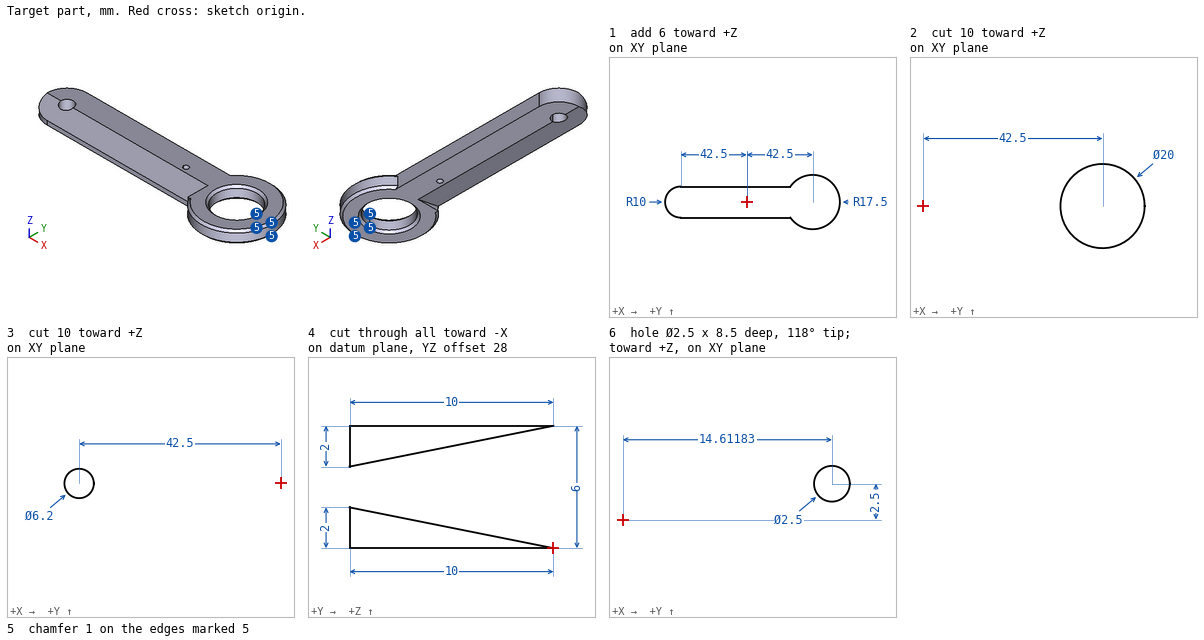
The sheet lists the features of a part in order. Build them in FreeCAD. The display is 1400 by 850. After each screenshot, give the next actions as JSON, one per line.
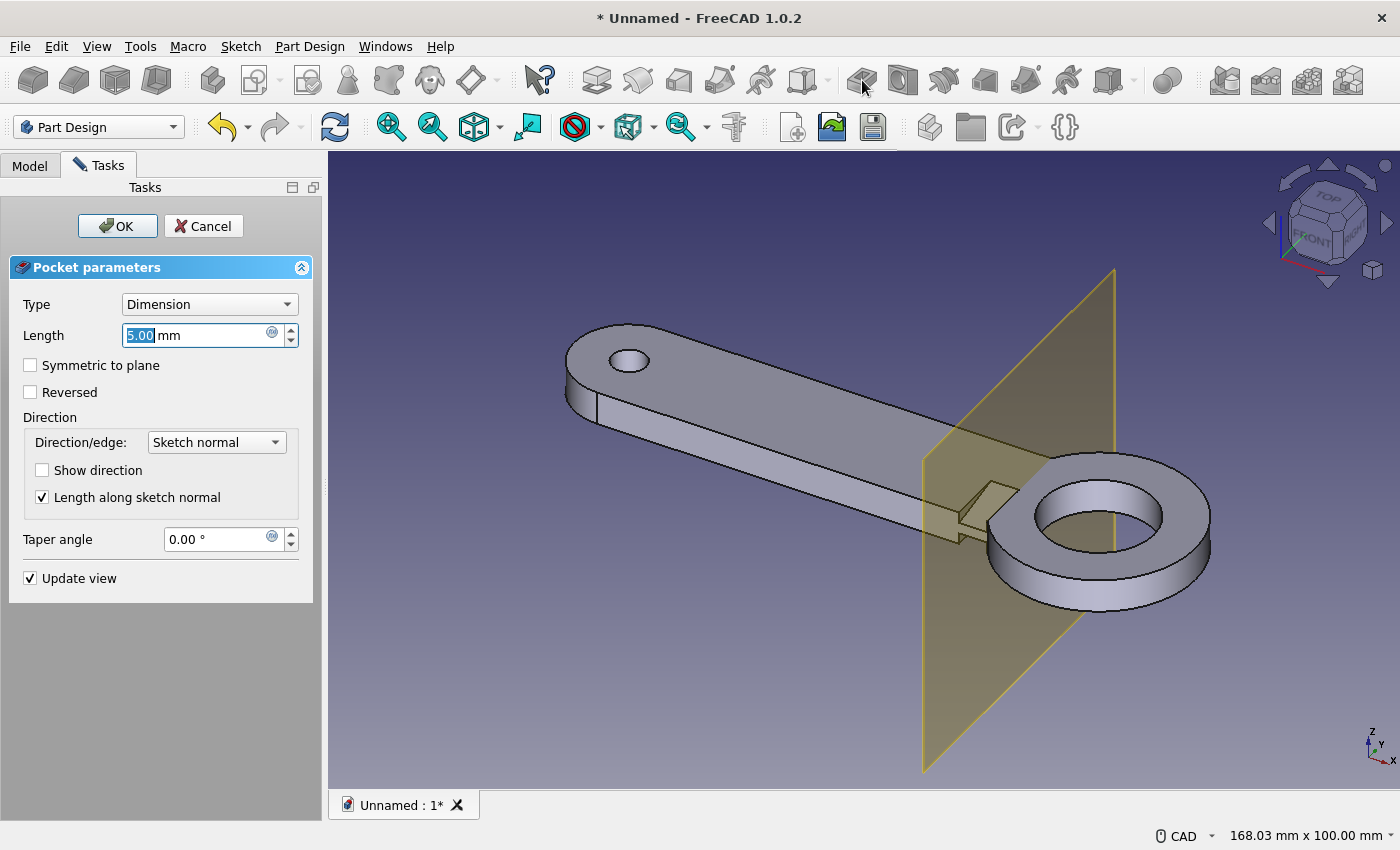
{"action": "left_click", "coordinate": [210, 304]}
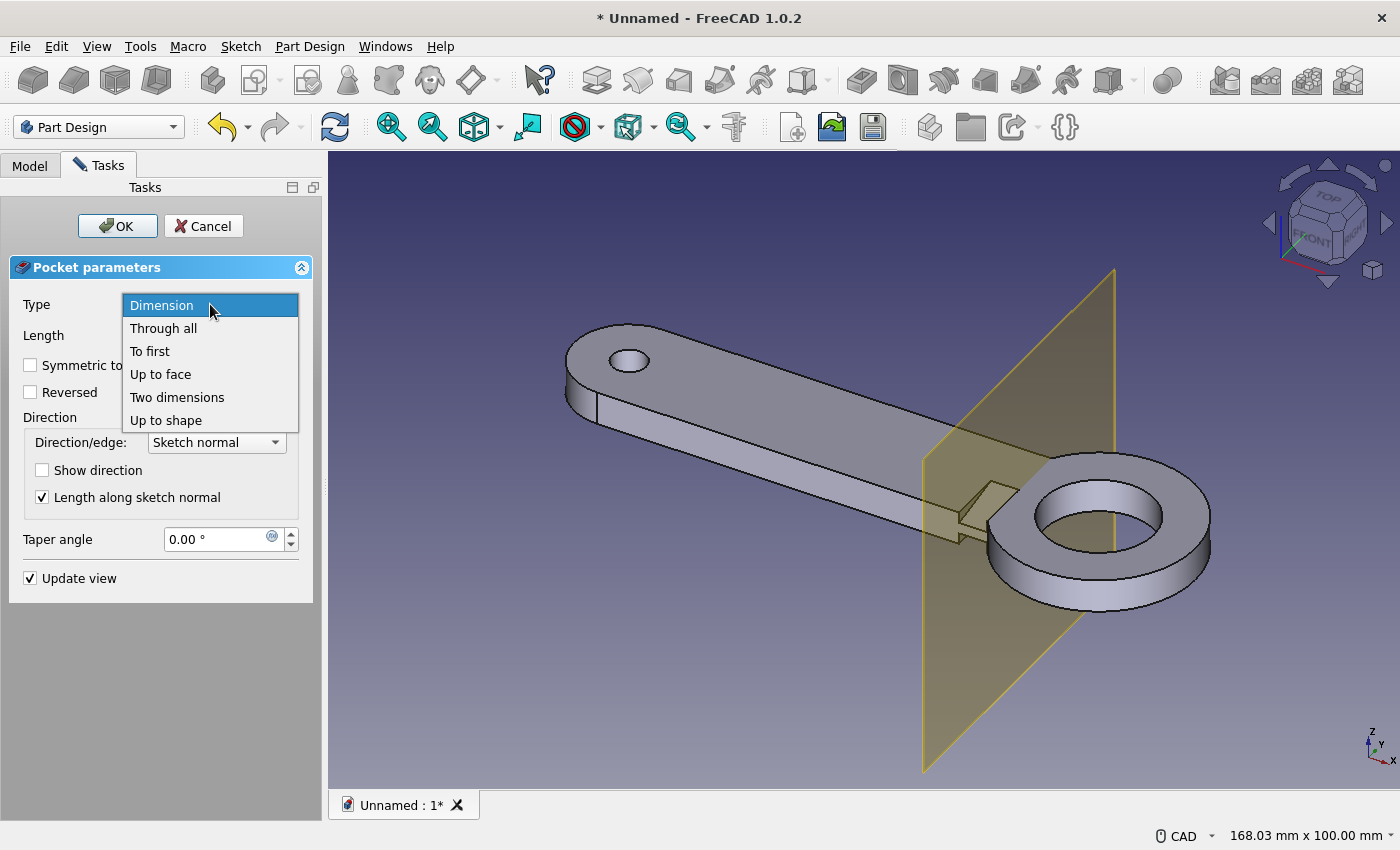
{"action": "left_click", "coordinate": [208, 328]}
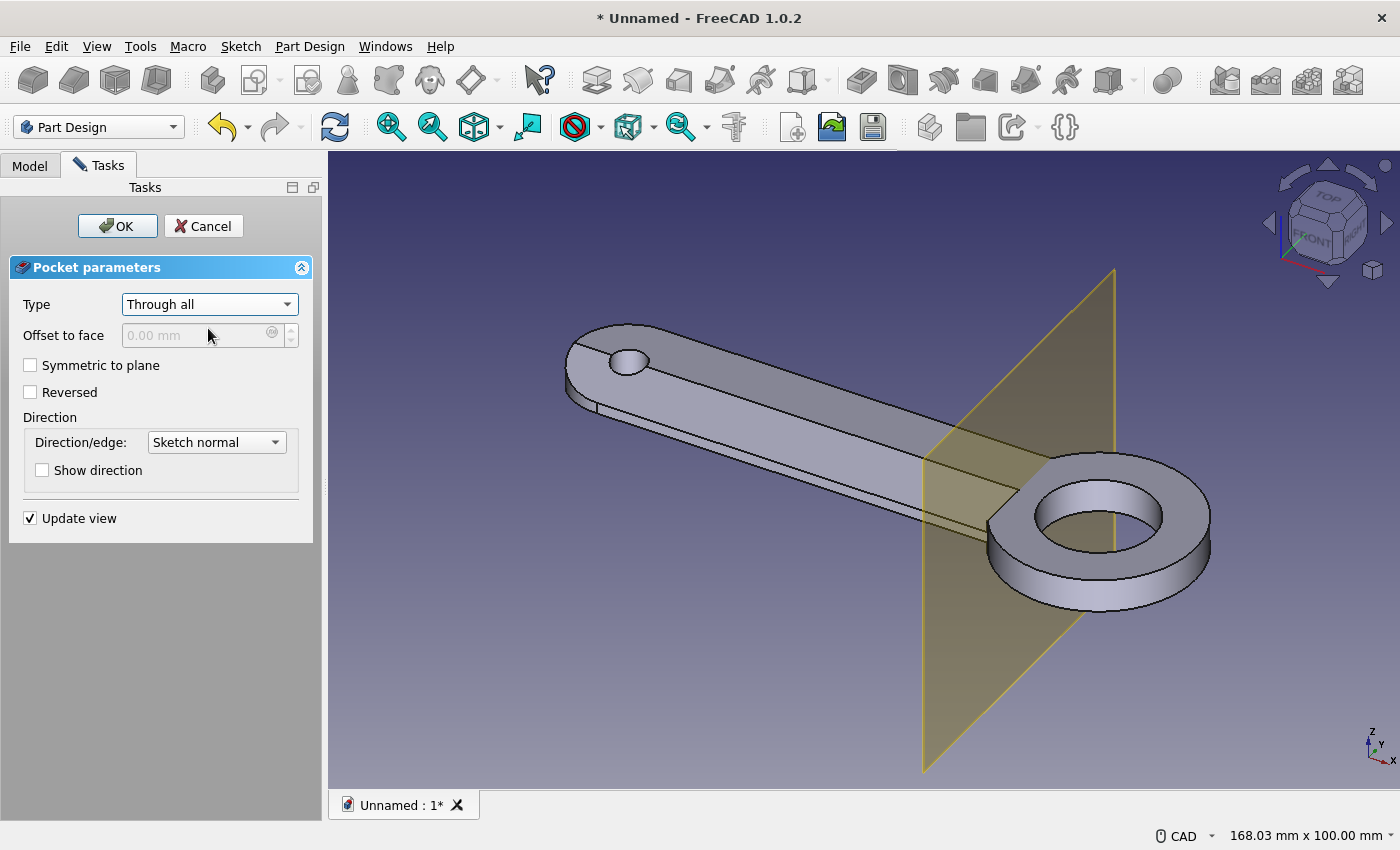
{"action": "left_click", "coordinate": [118, 226]}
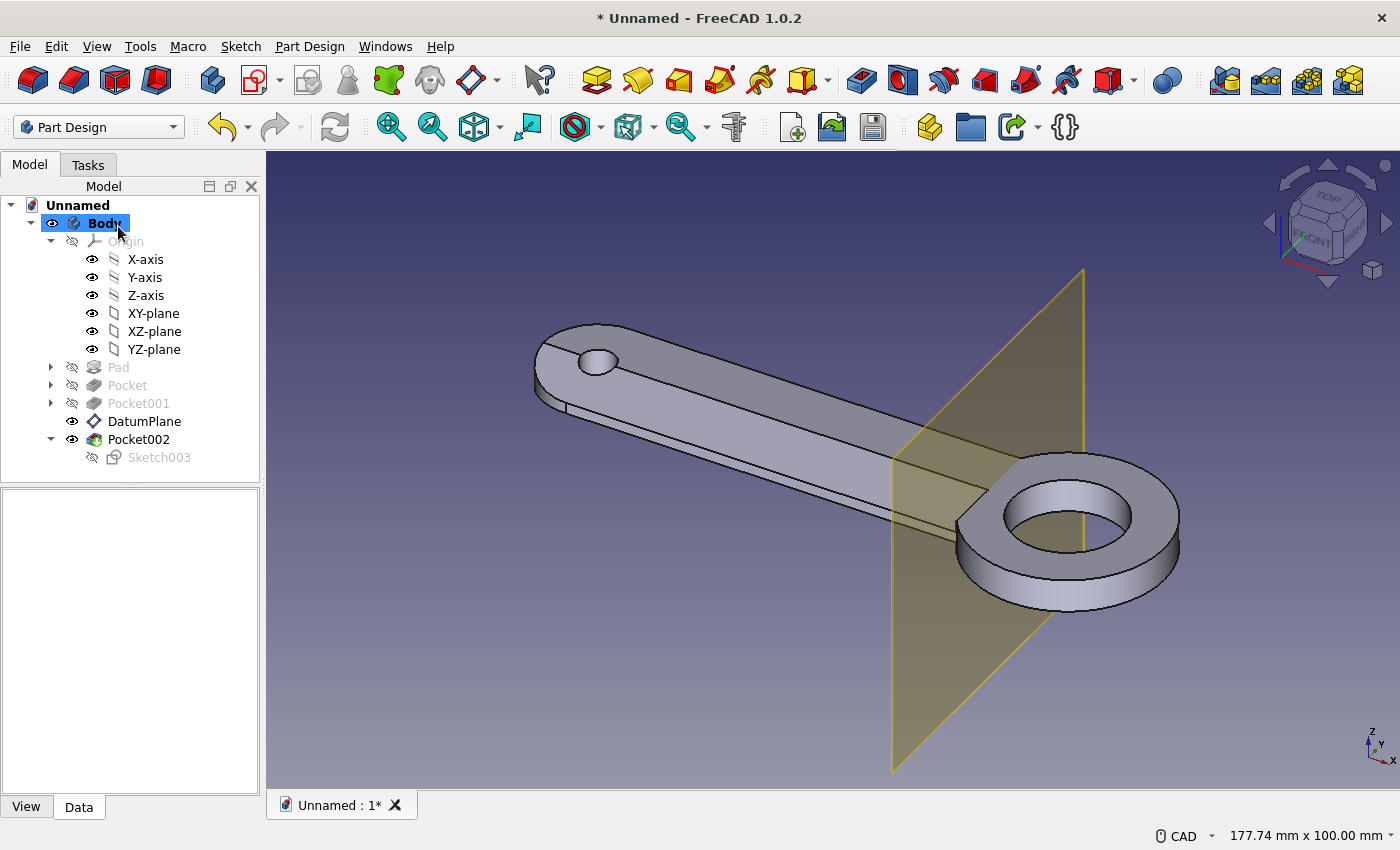
{"action": "left_click", "coordinate": [117, 421]}
{"action": "key", "text": "space"}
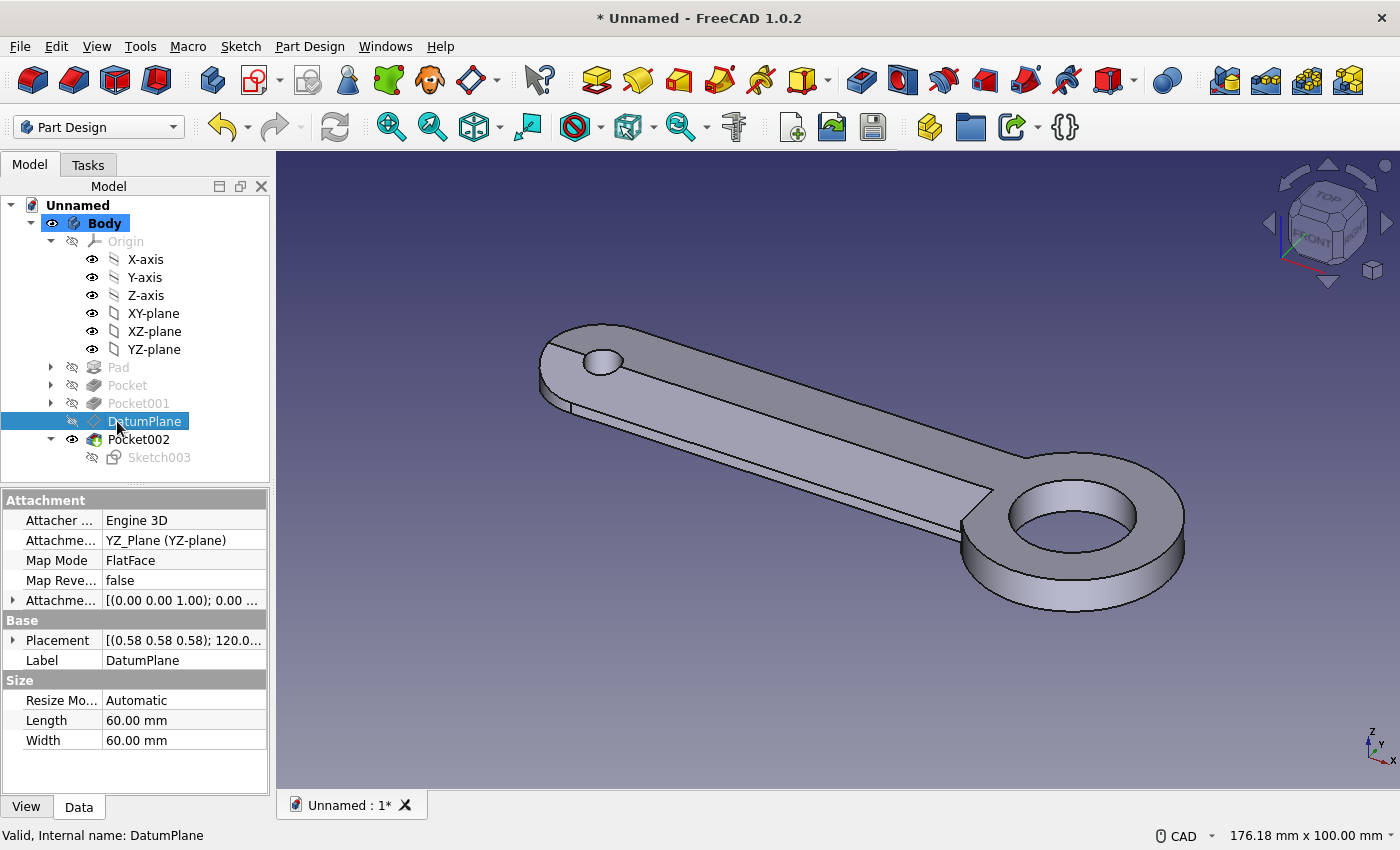
{"action": "left_click", "coordinate": [1170, 547]}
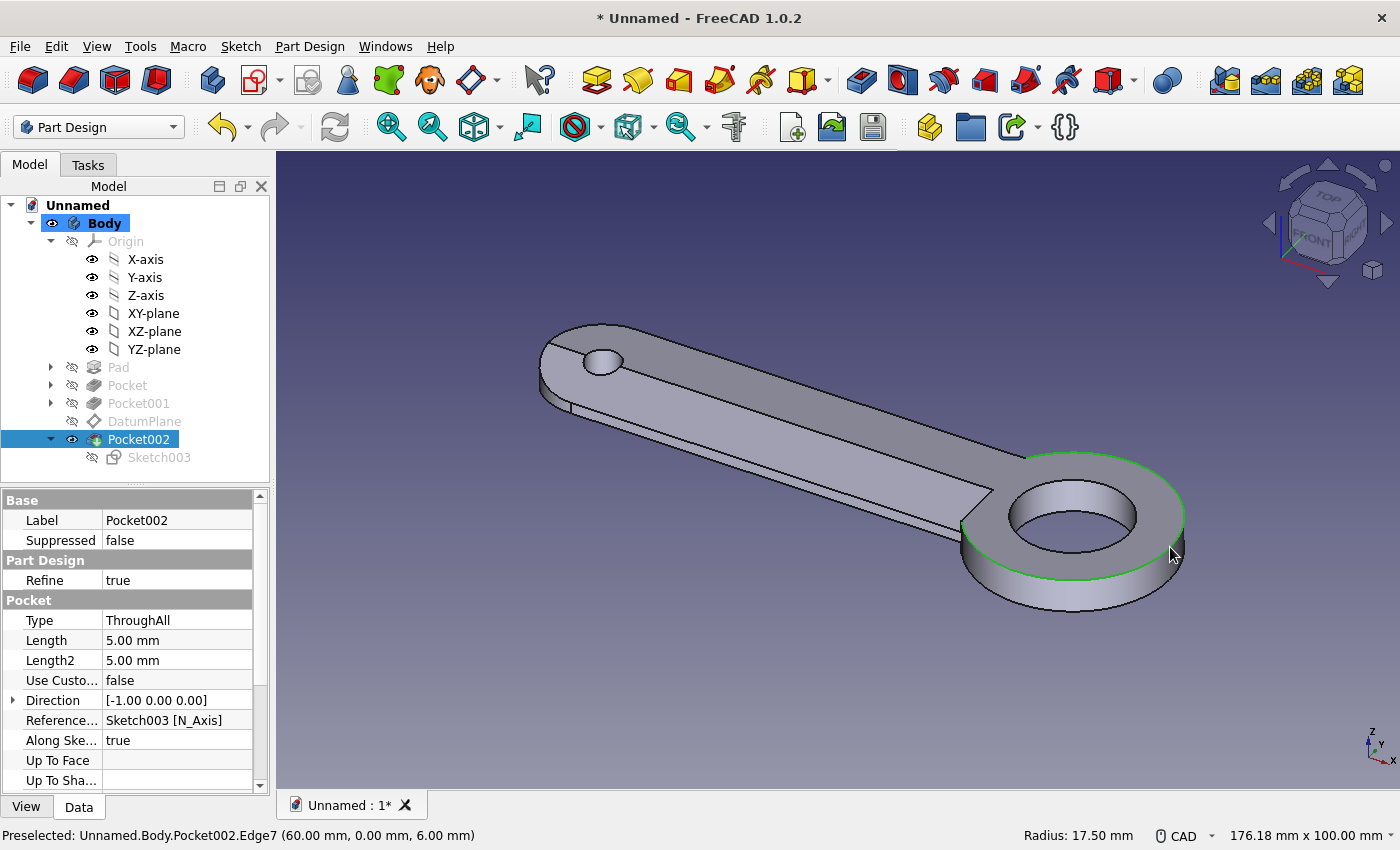
{"action": "left_click", "coordinate": [1018, 497], "text": "ctrl"}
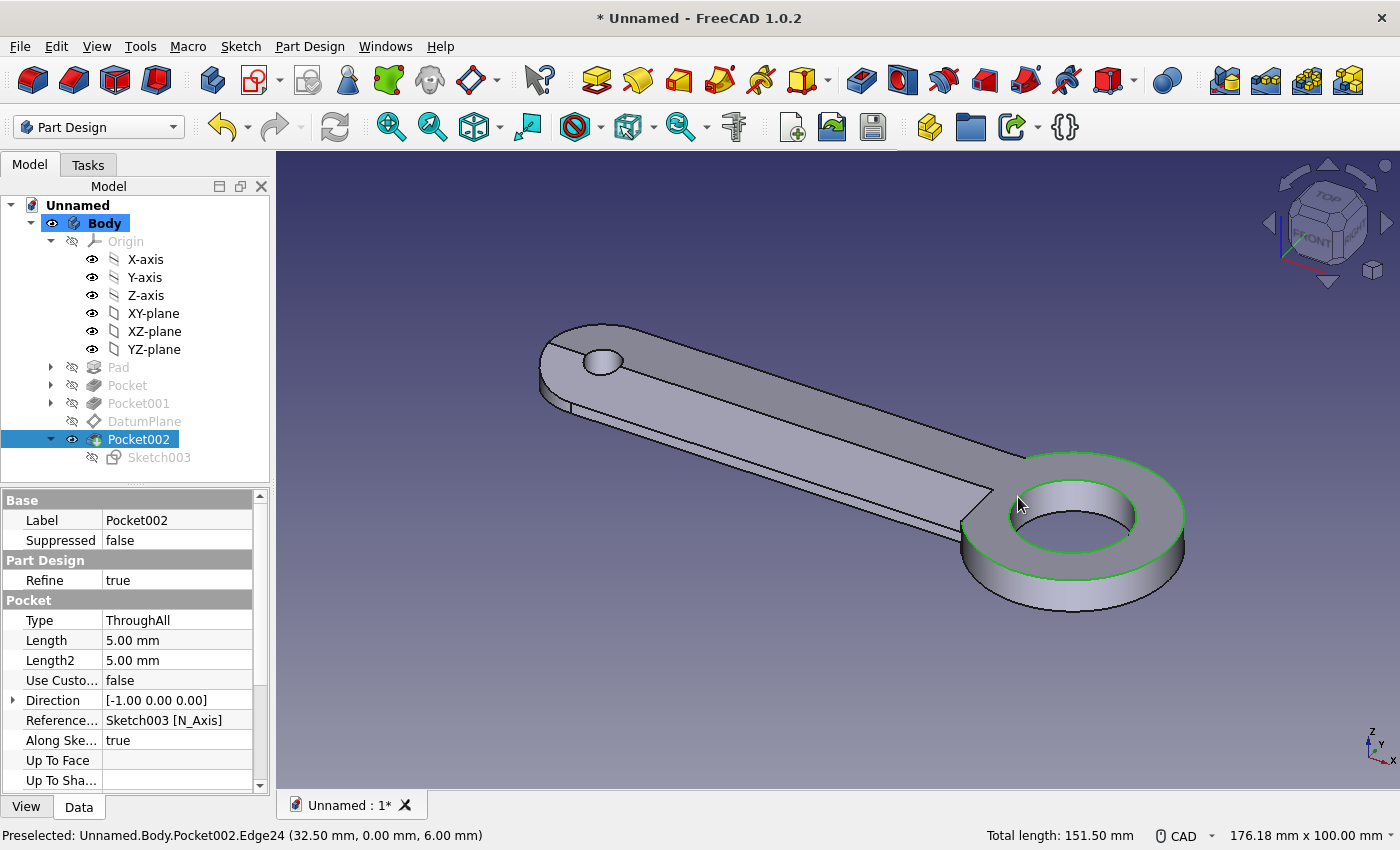
{"action": "left_click", "coordinate": [1022, 604], "text": "ctrl"}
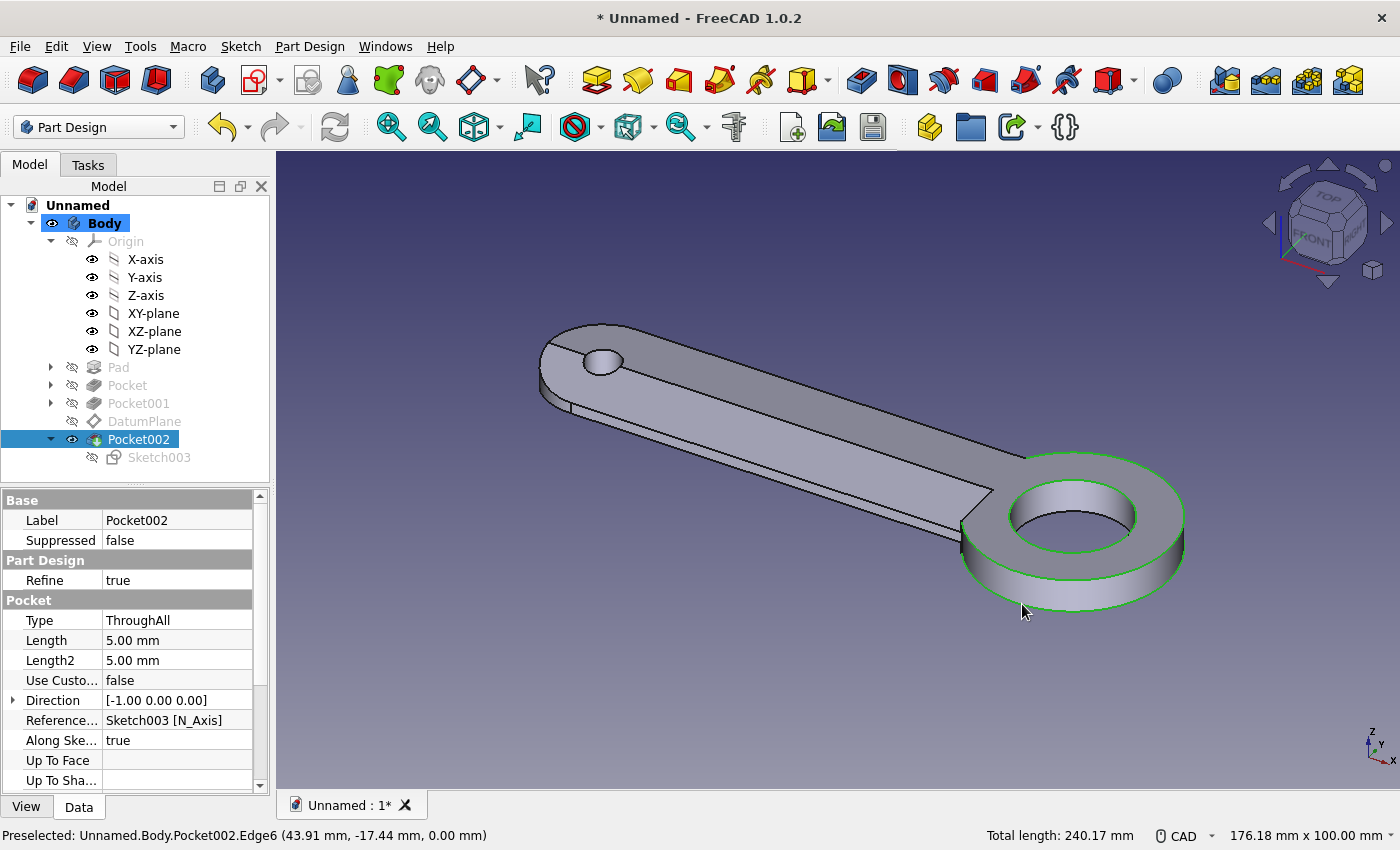
{"action": "key", "text": "0"}